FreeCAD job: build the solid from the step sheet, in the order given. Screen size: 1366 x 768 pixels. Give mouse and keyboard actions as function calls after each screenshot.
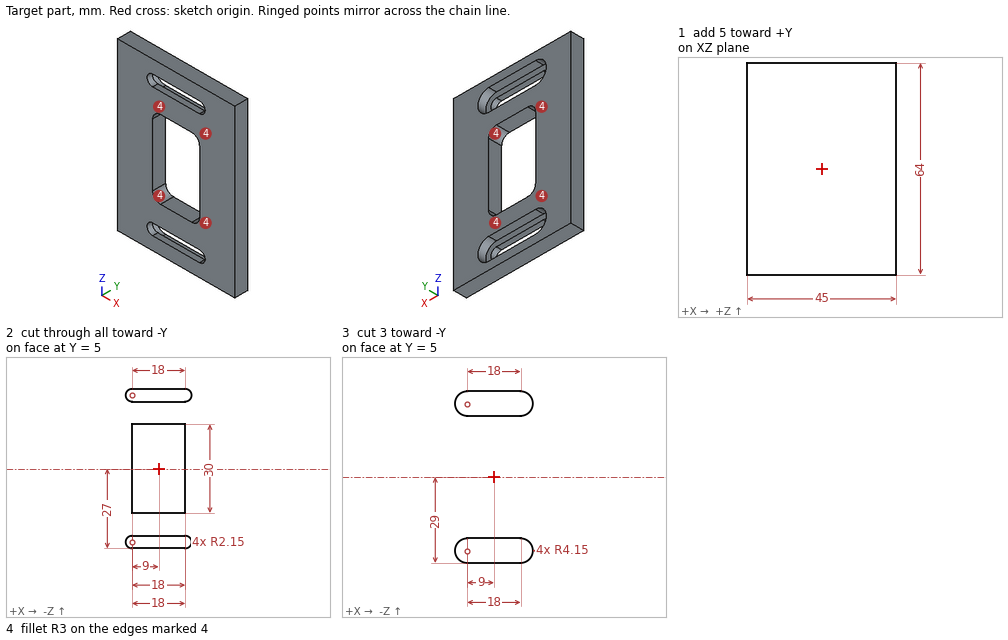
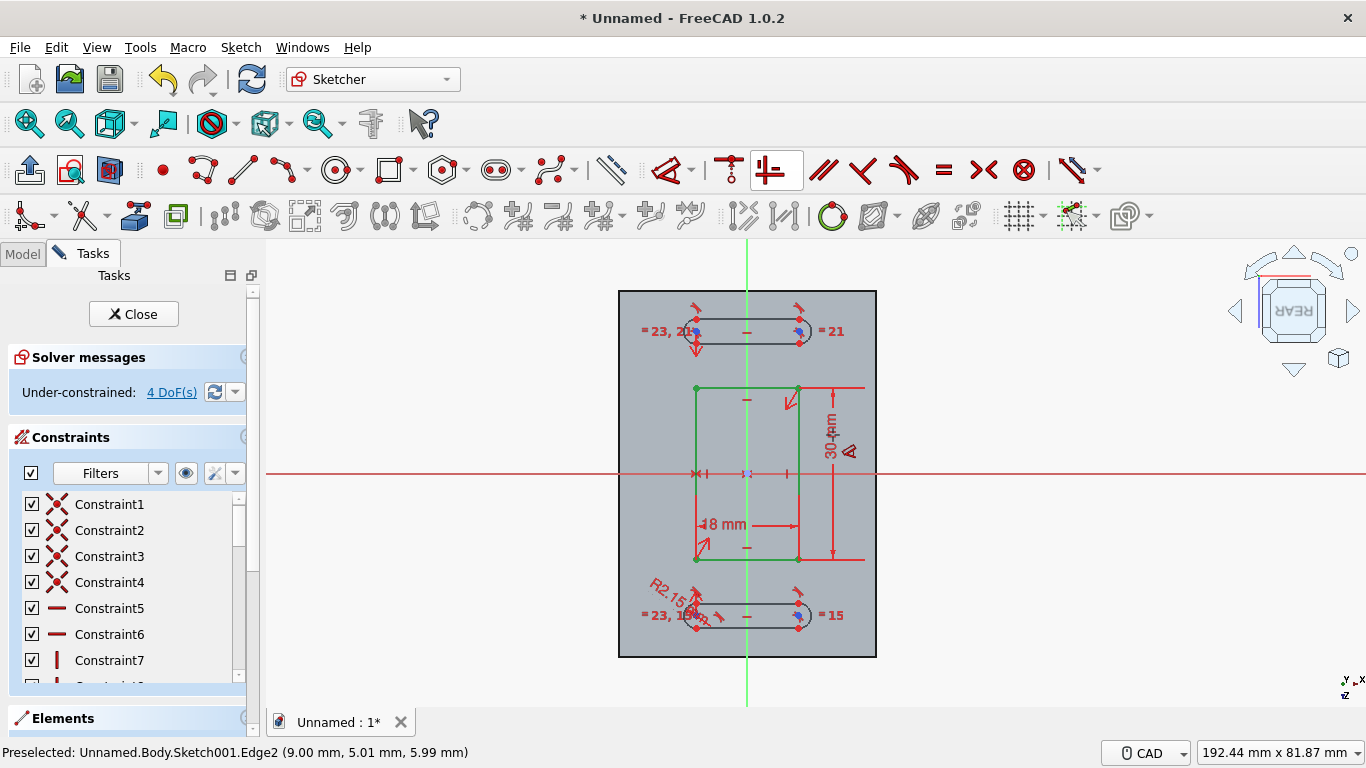
click(727, 604)
click(724, 662)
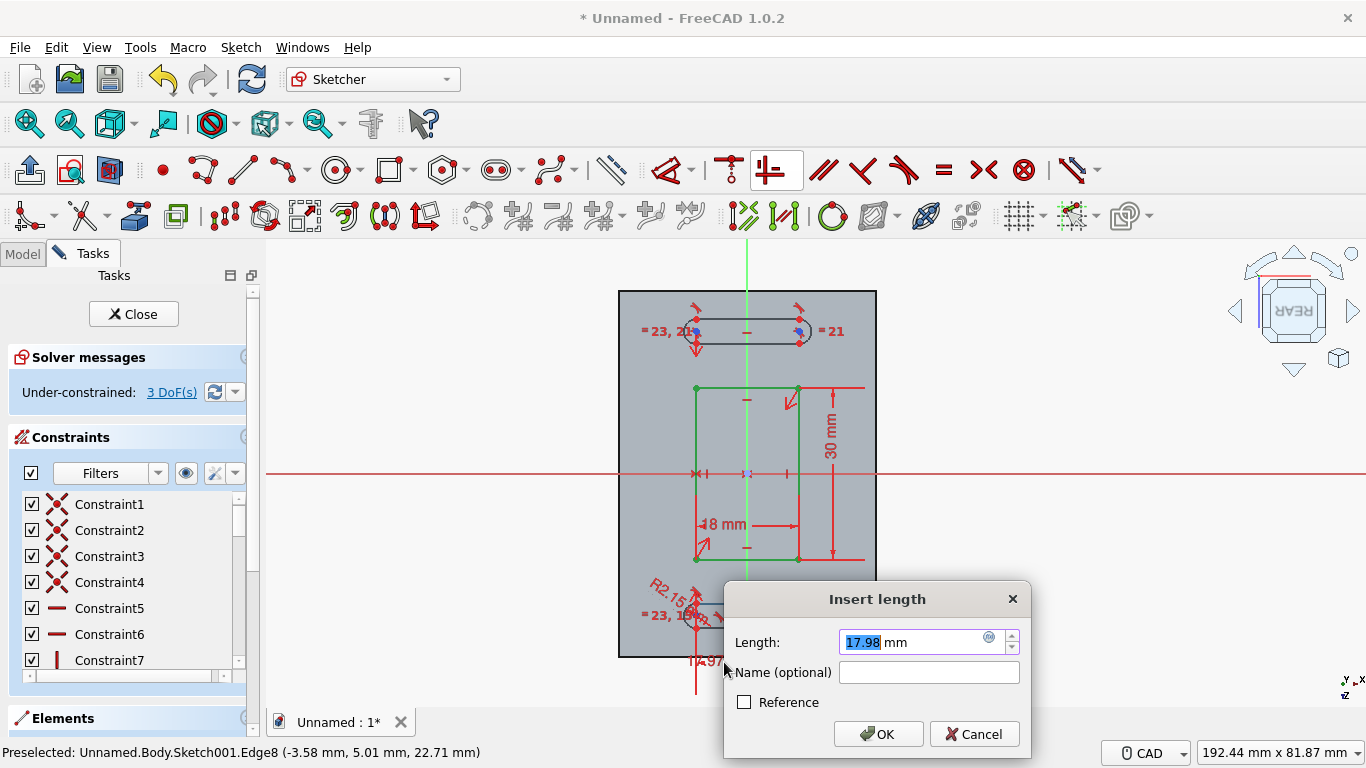
text(18)
key(Return)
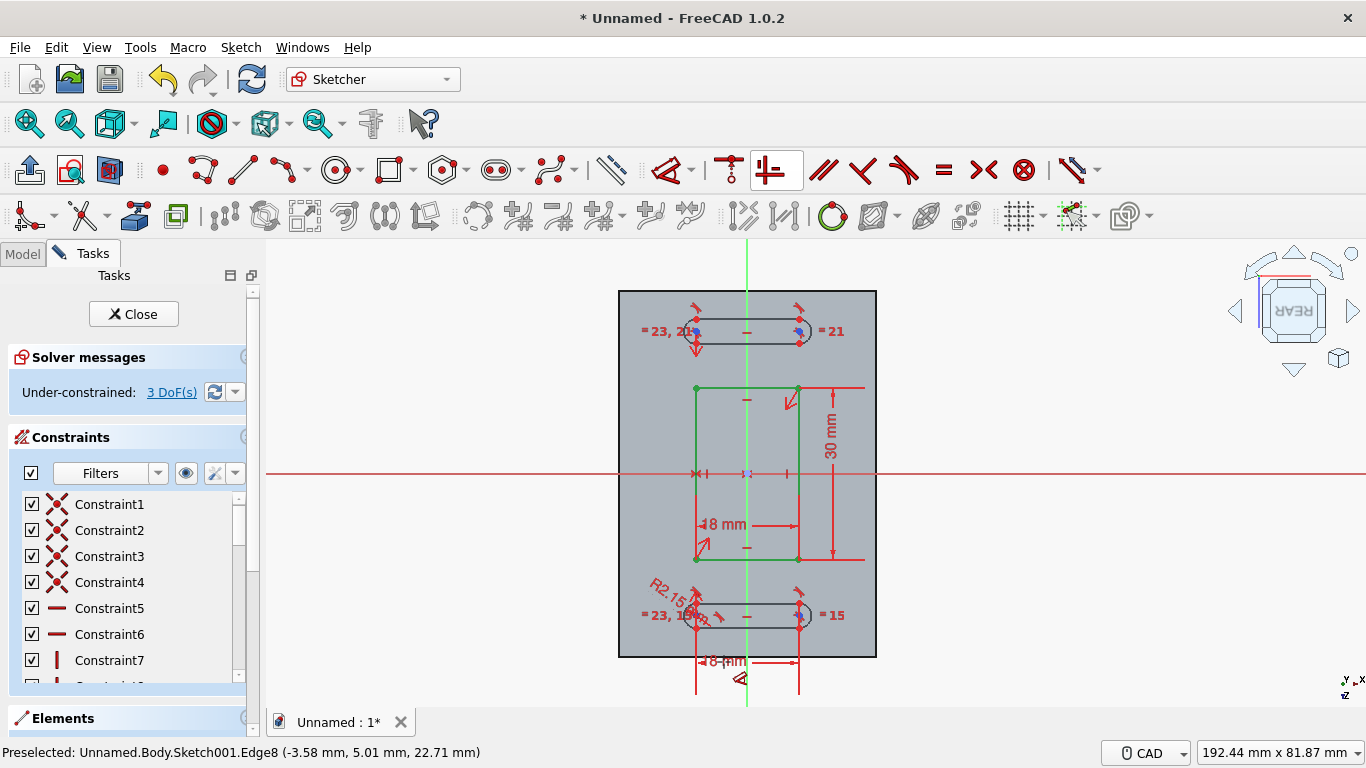
click(727, 319)
click(724, 285)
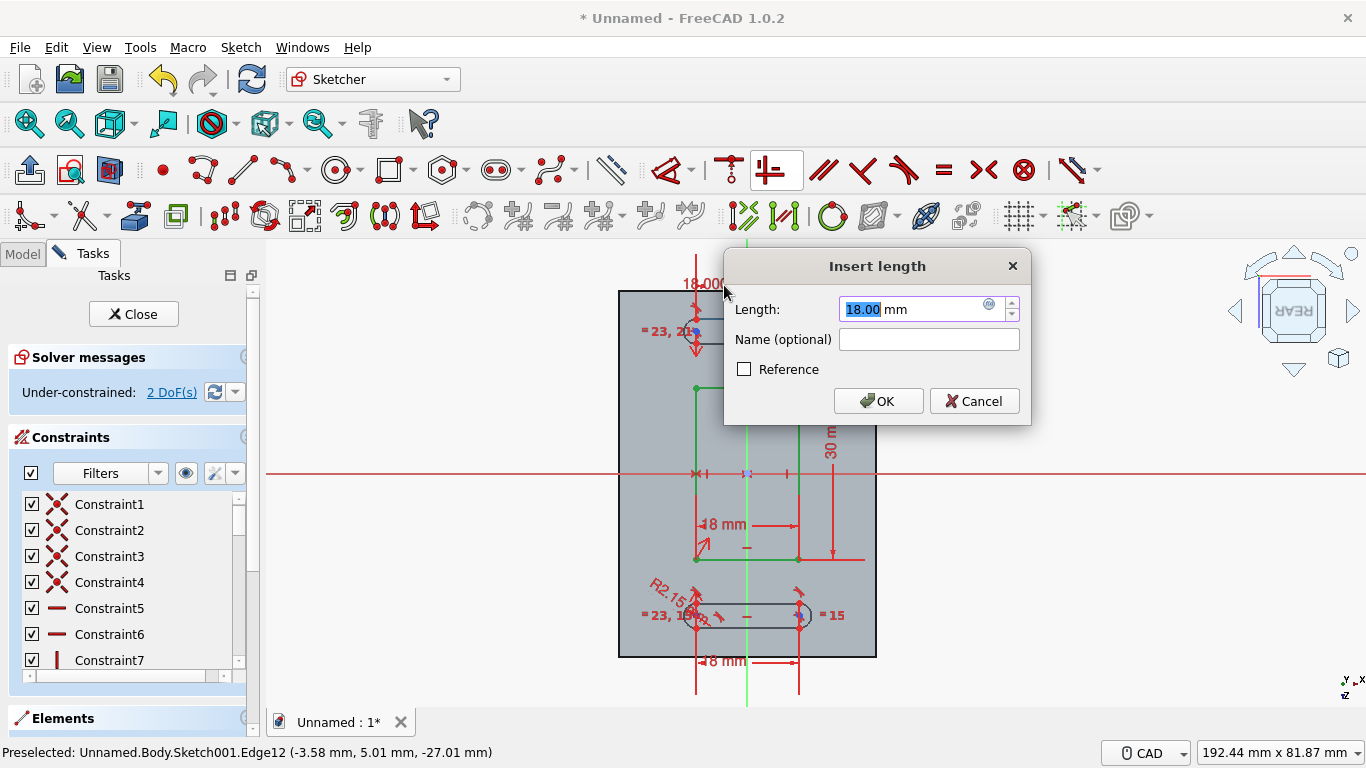
text(18)
key(Return)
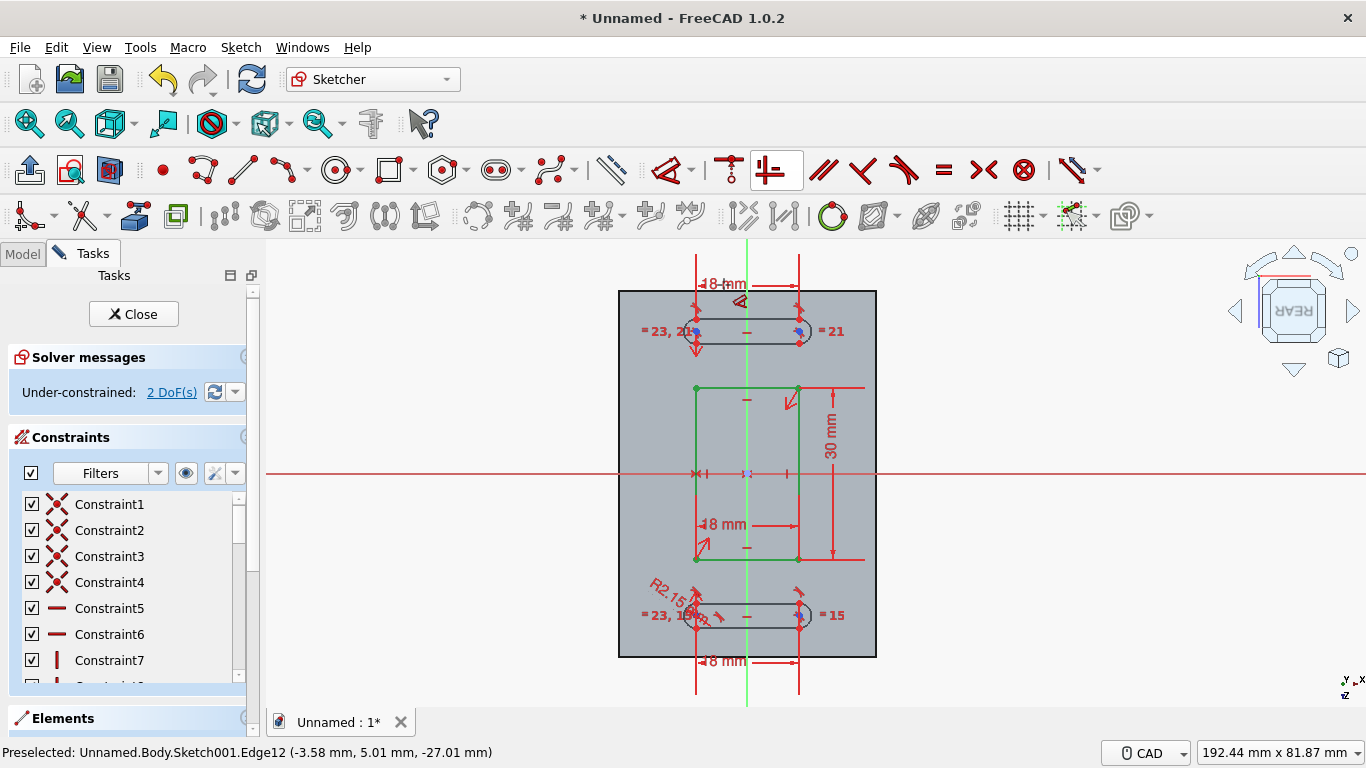
click(696, 604)
click(722, 440)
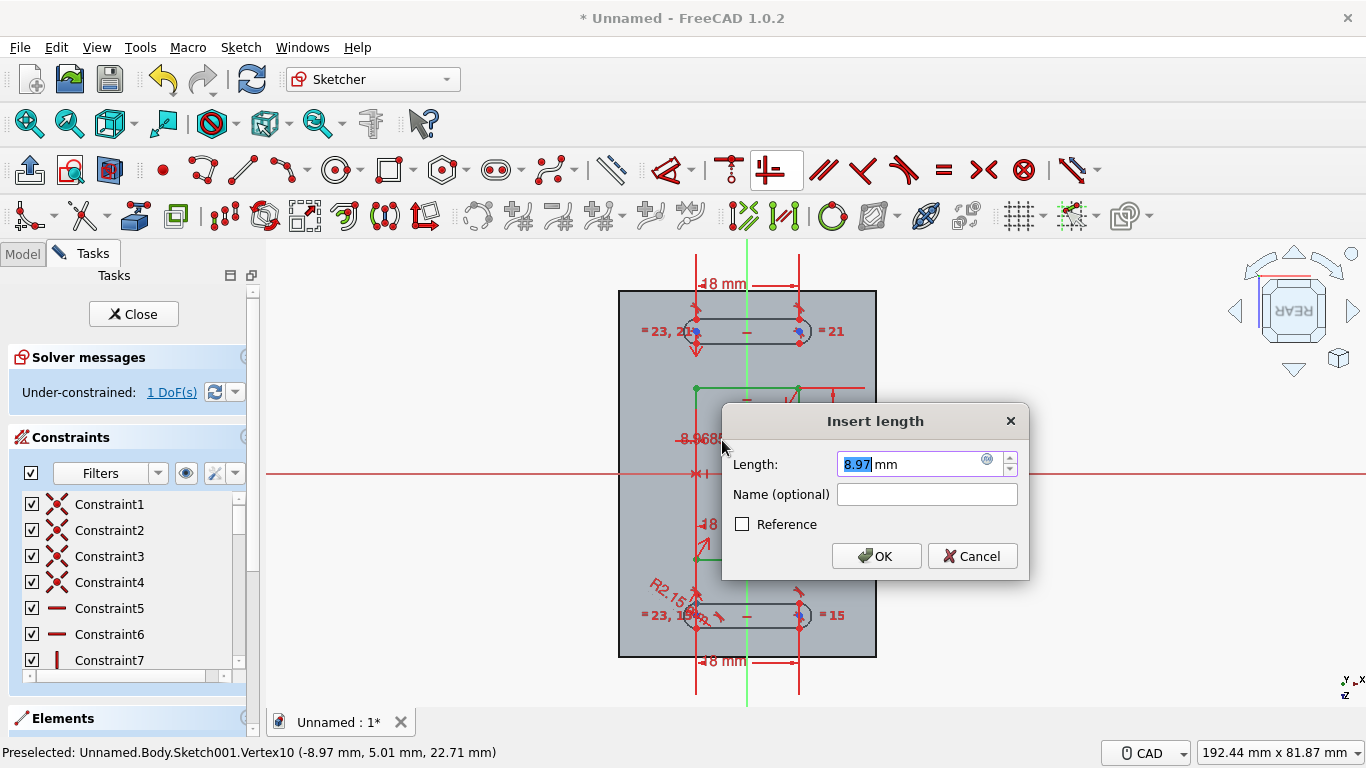
text(9)
key(Return)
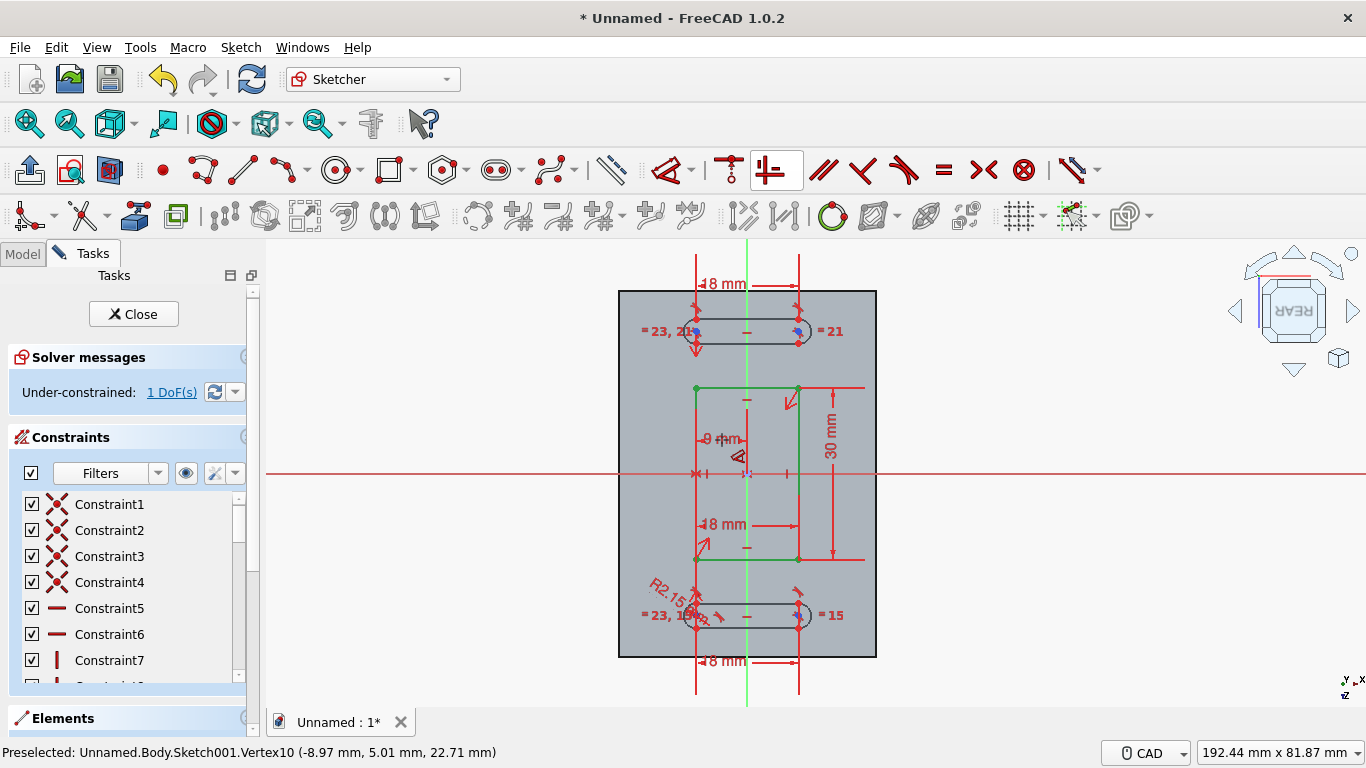
click(696, 628)
click(662, 551)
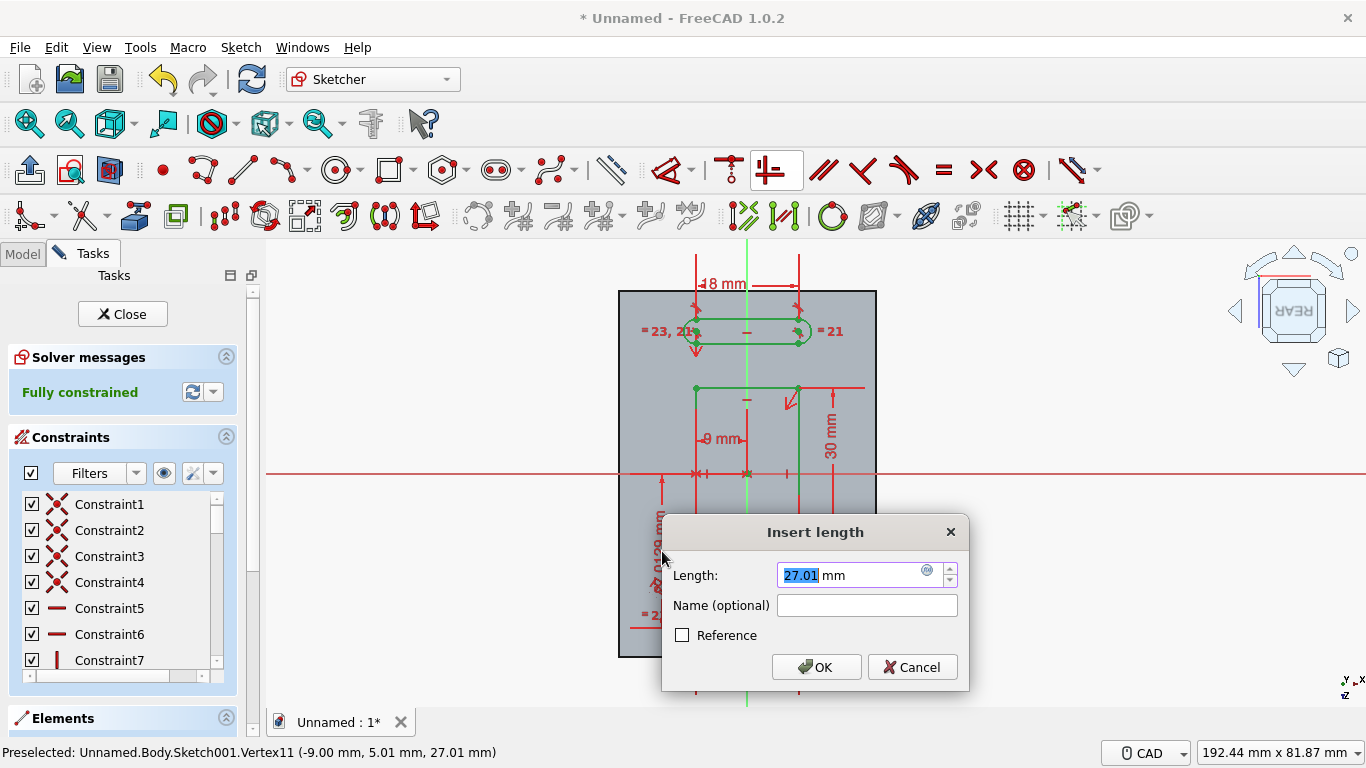
text(27)
key(Return)
key(Escape)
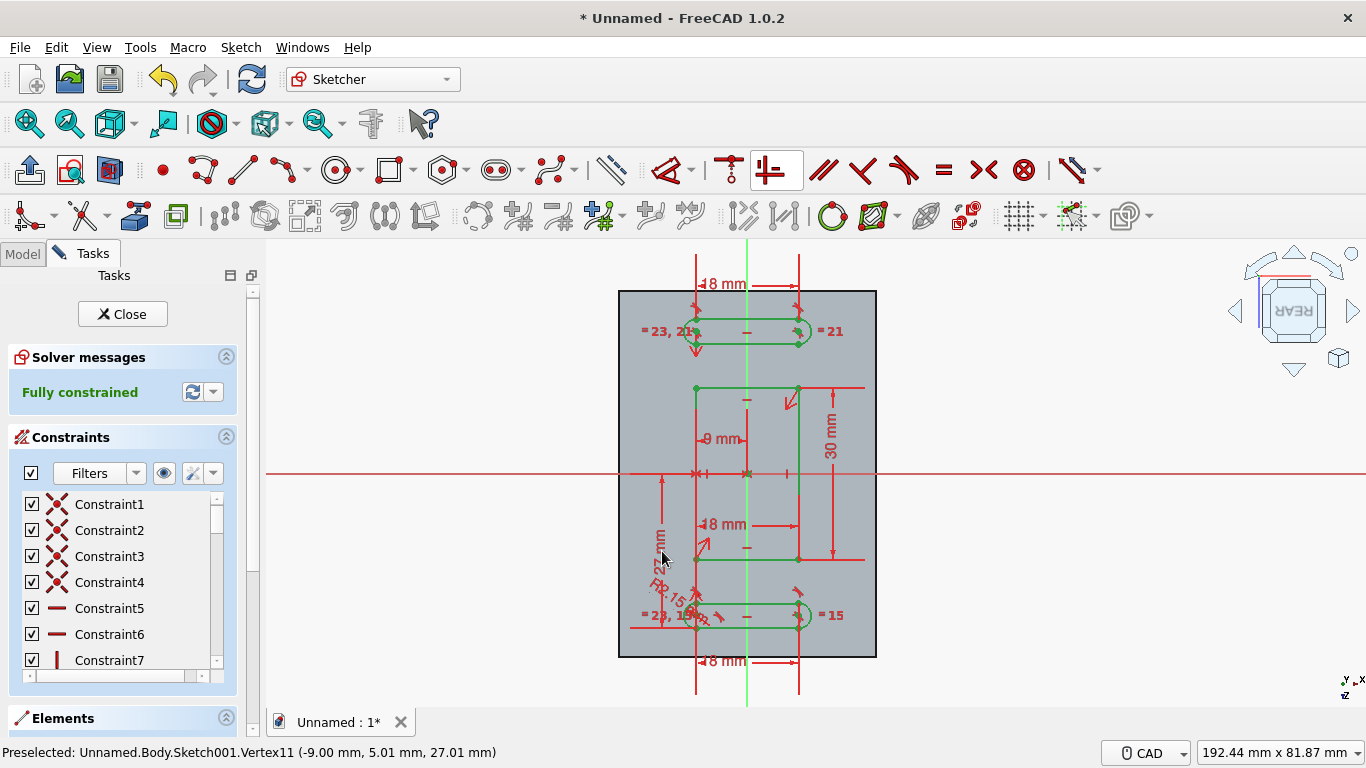
click(123, 314)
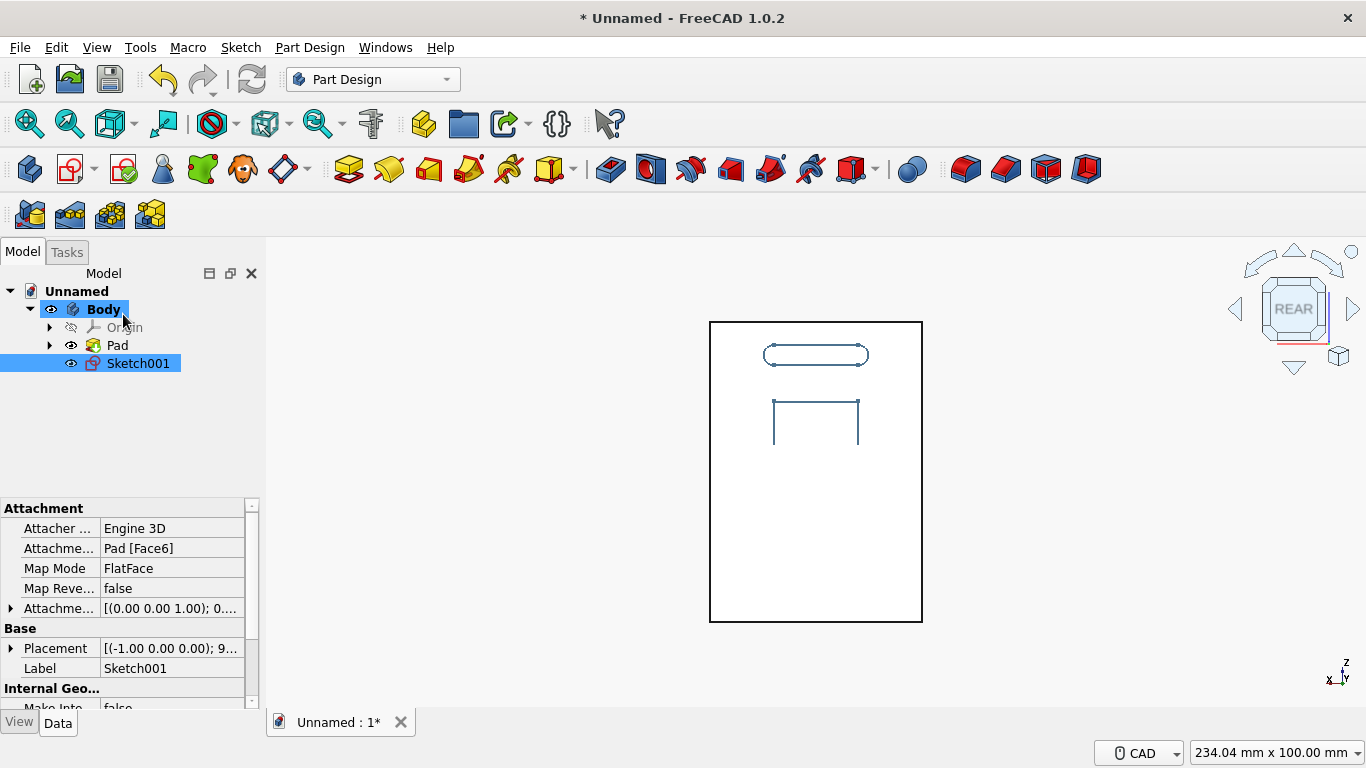
click(612, 170)